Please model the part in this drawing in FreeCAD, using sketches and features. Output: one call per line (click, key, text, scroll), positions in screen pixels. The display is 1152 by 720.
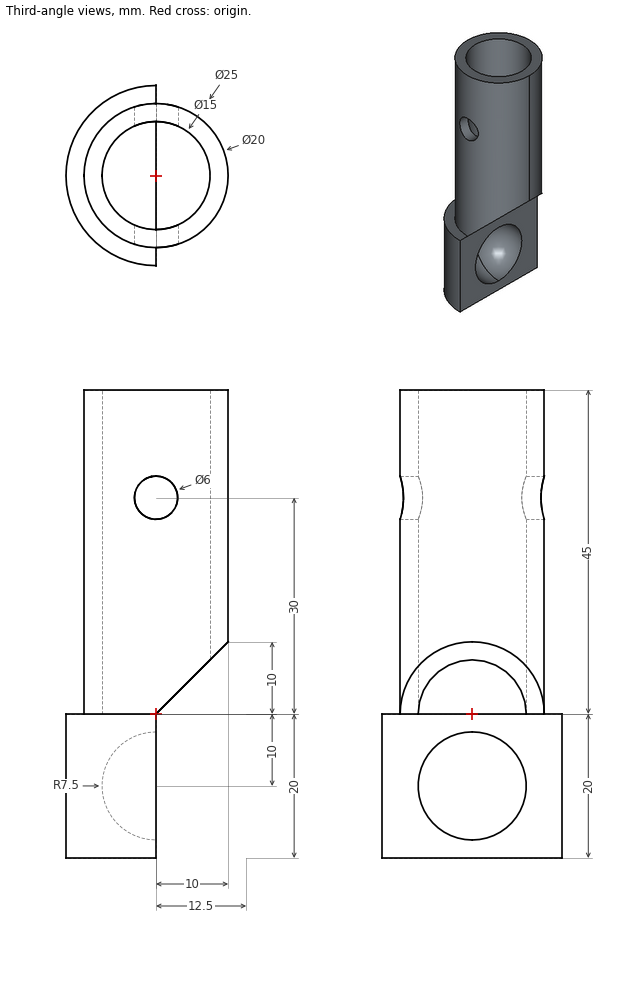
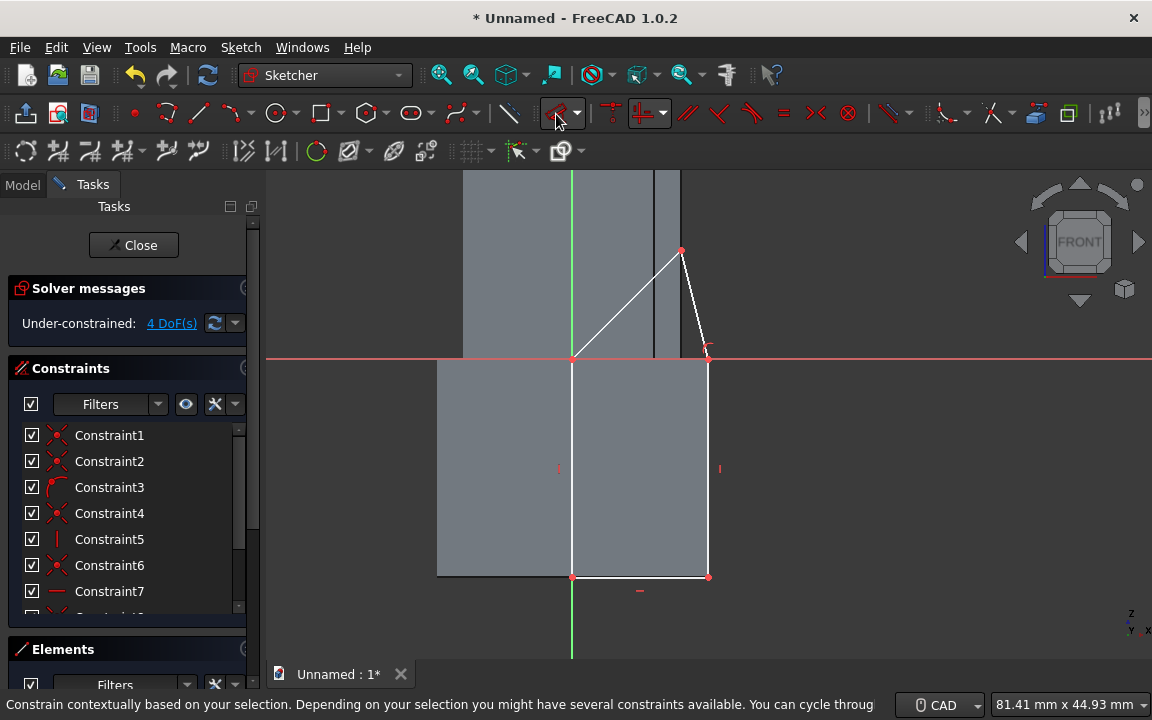
click(708, 425)
click(742, 469)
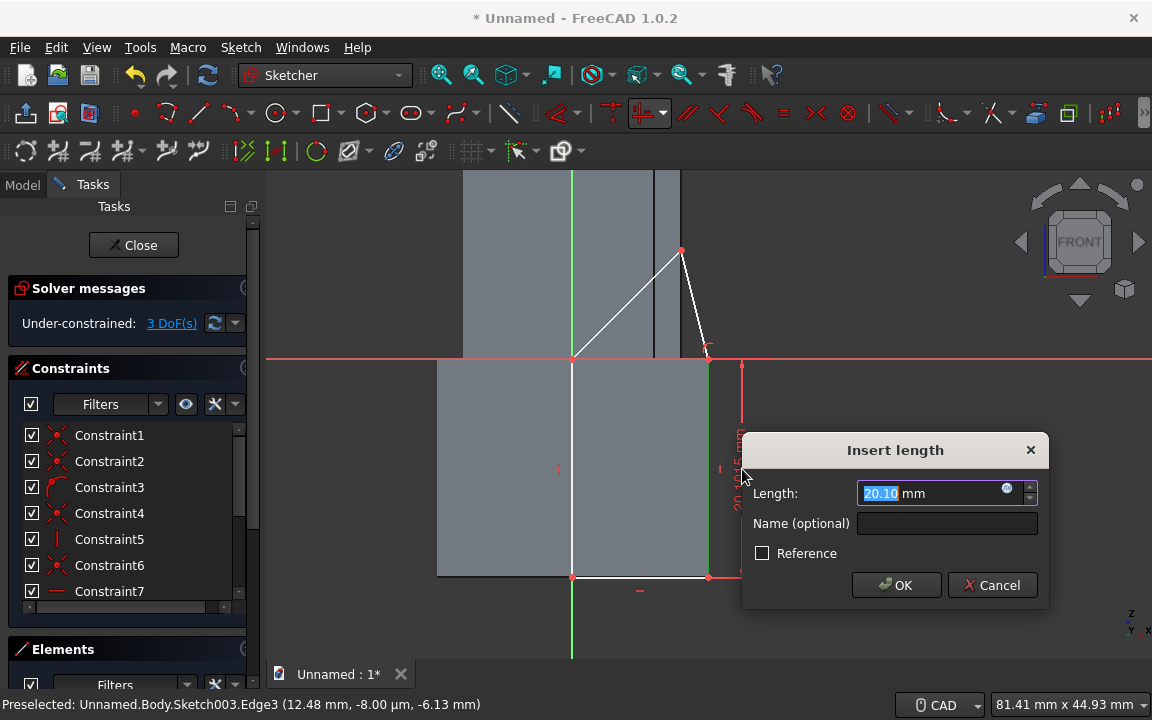
text(20)
key(Return)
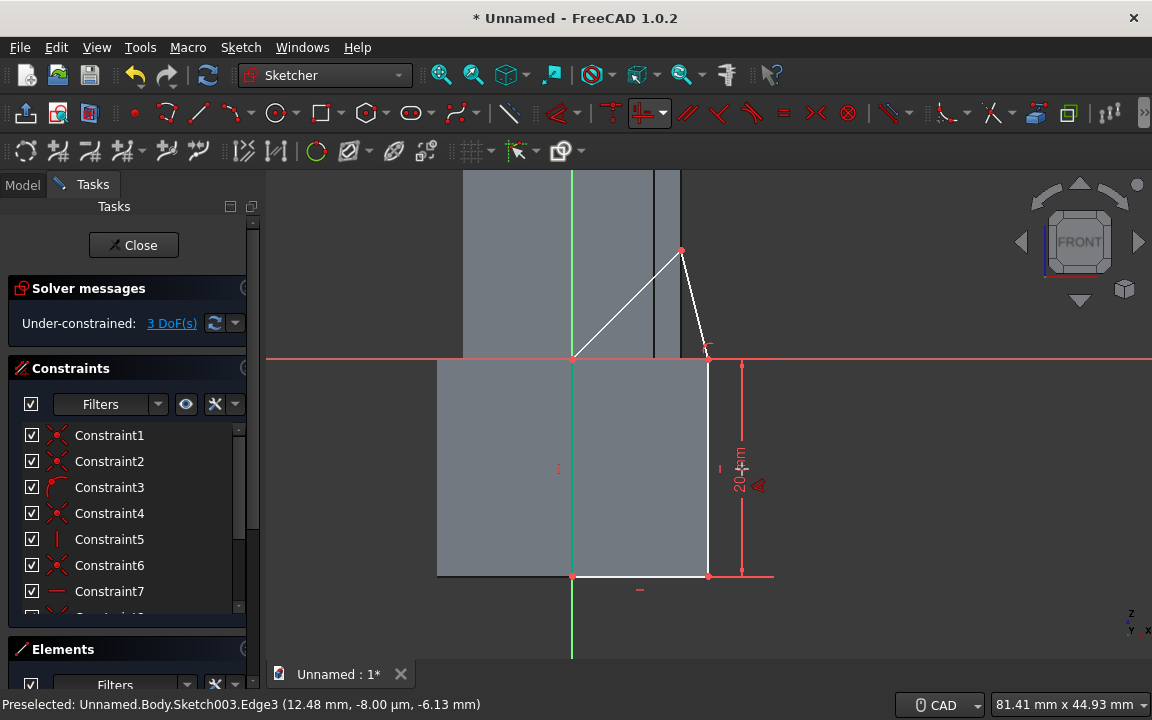
click(681, 251)
click(627, 217)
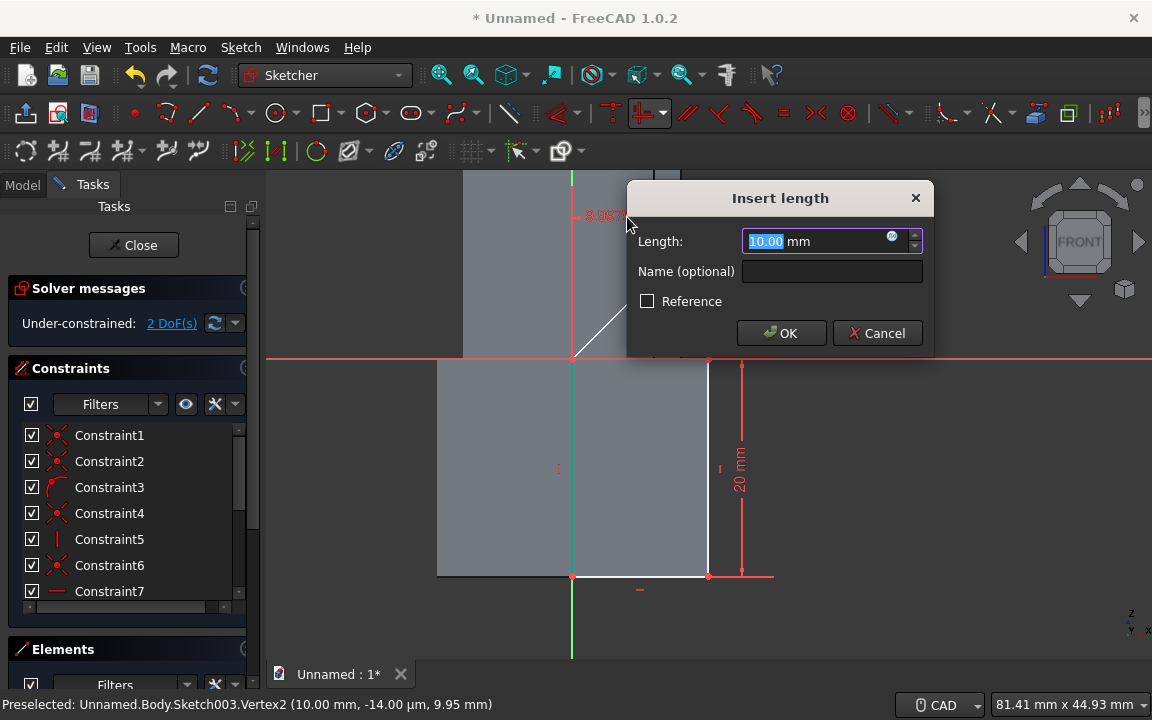
text(10)
key(Return)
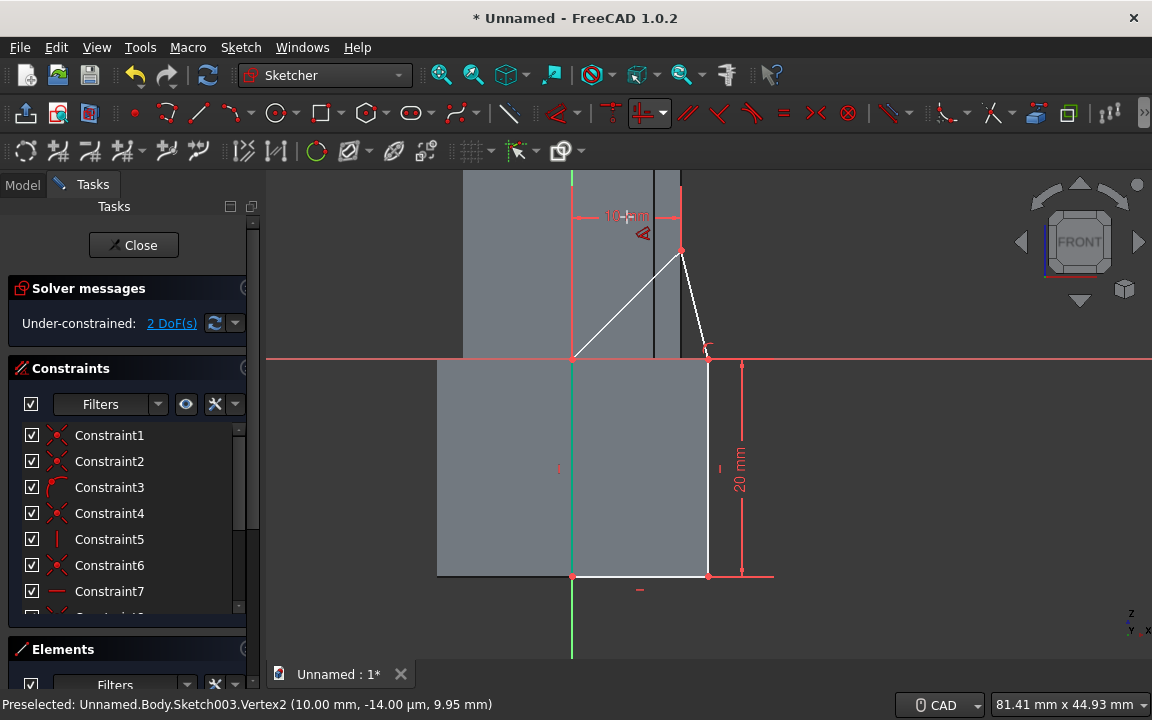
click(681, 251)
click(538, 305)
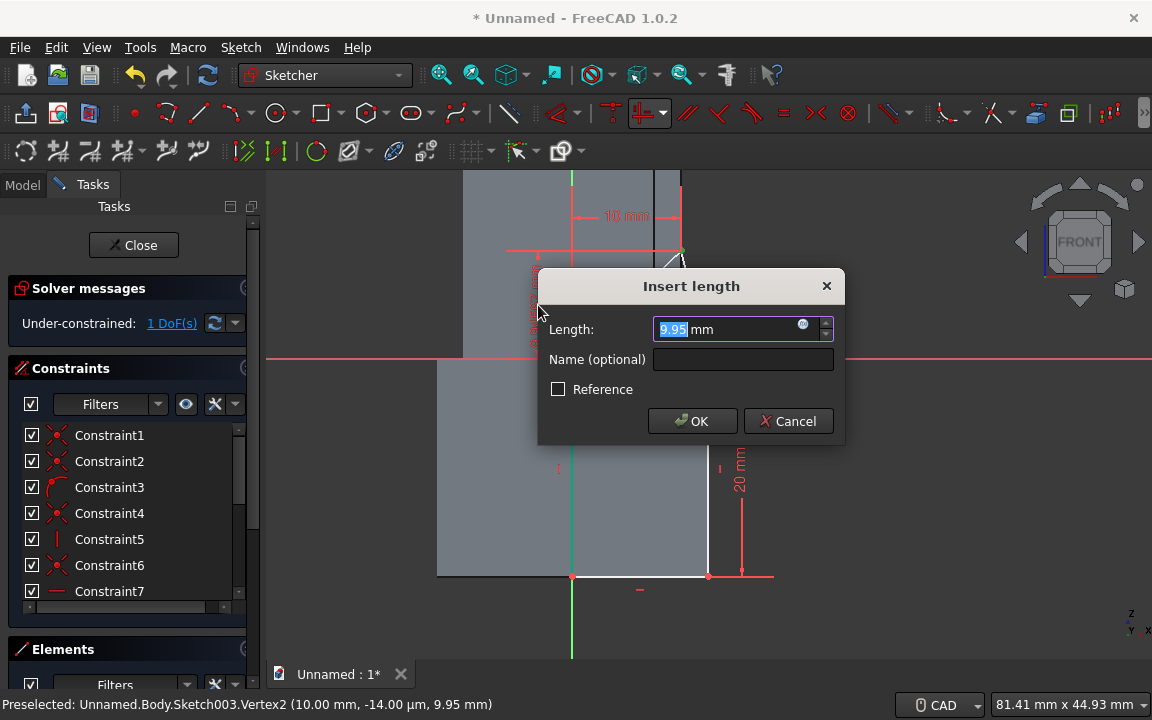
text(10)
key(Return)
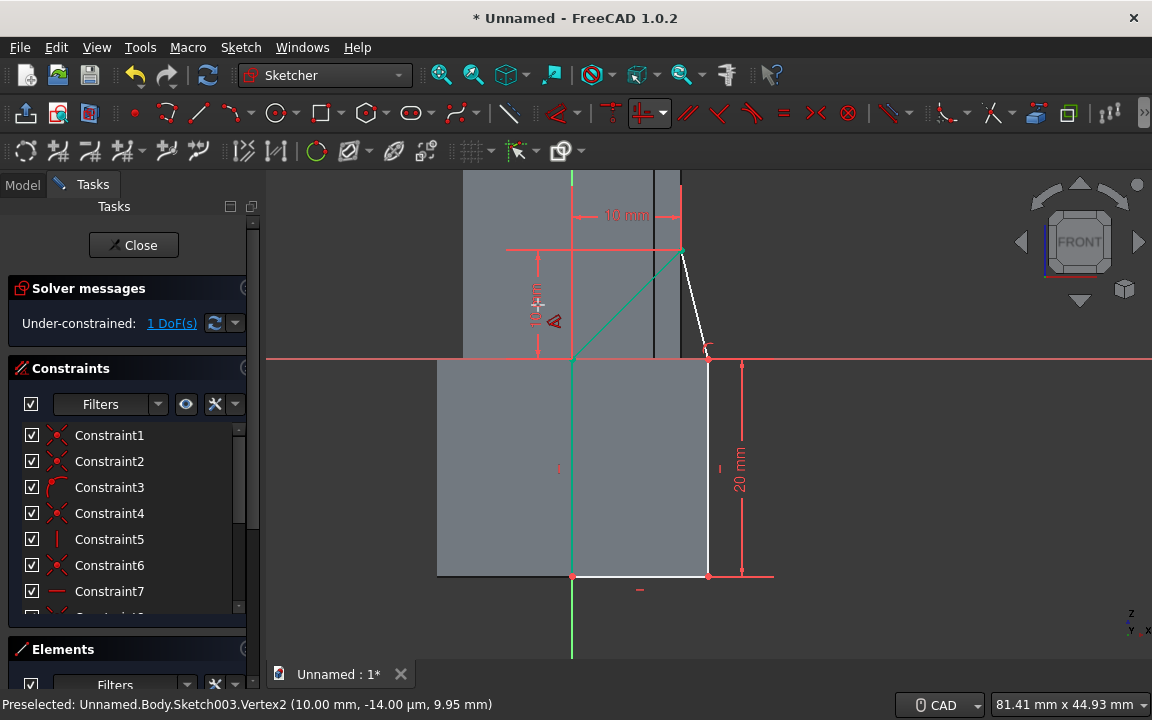
click(667, 577)
click(640, 611)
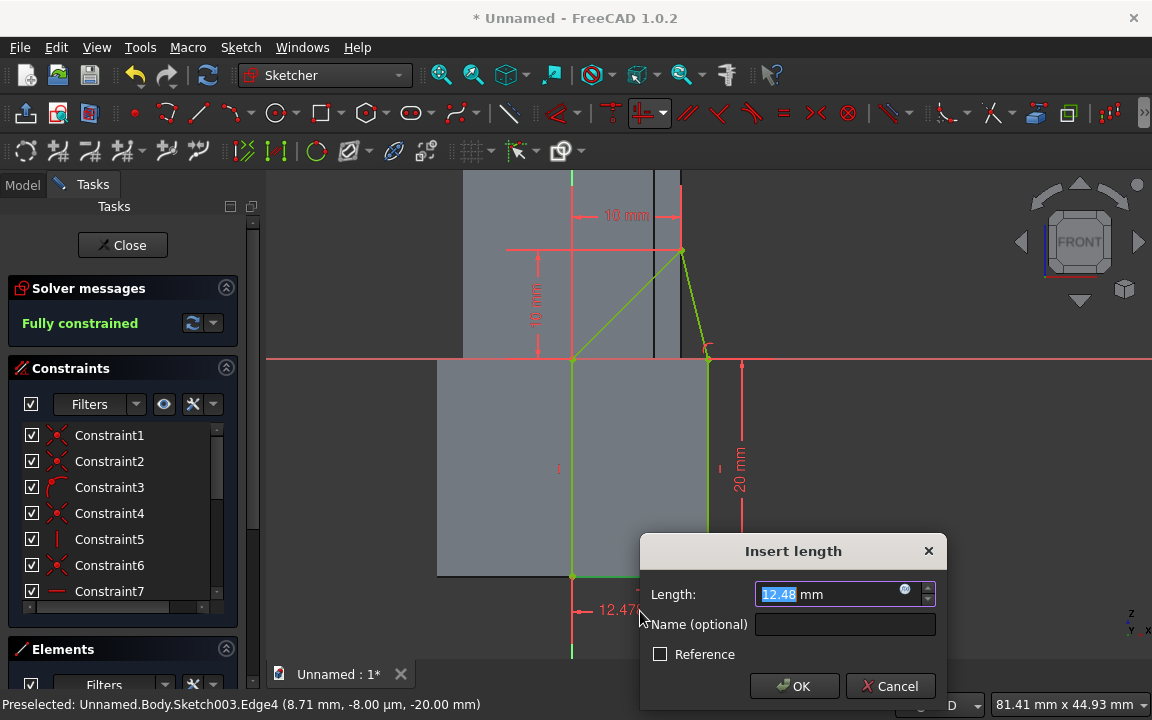
text(12.5)
key(Return)
key(Escape)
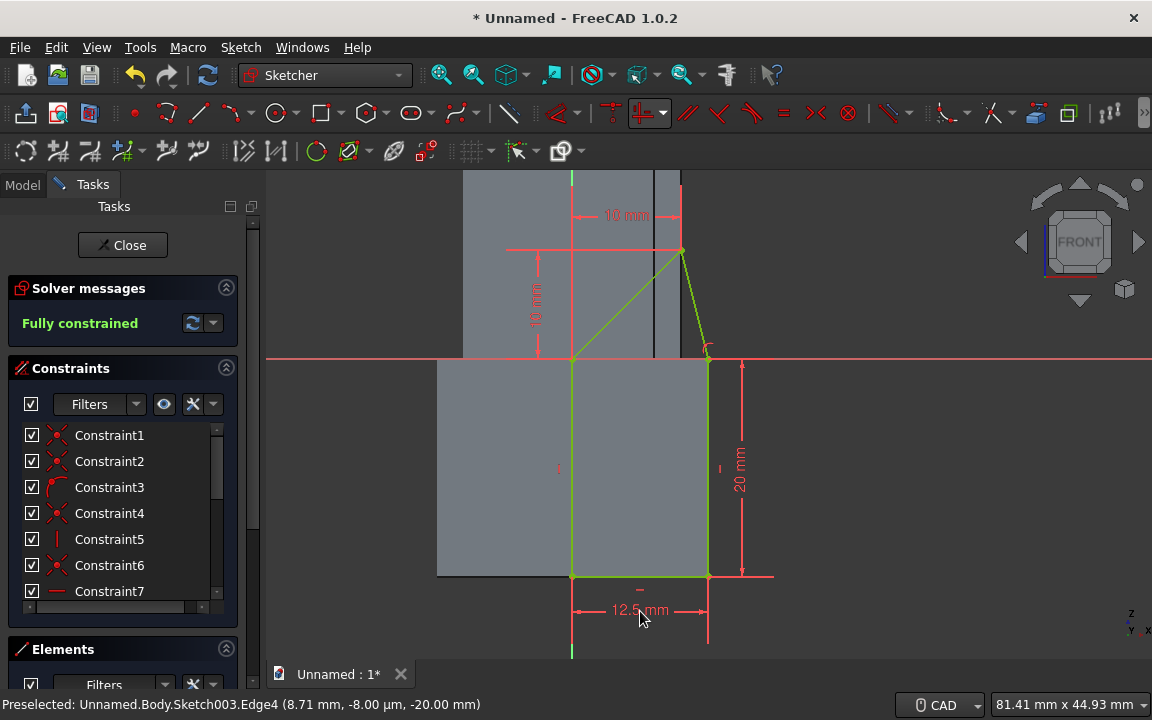
click(123, 245)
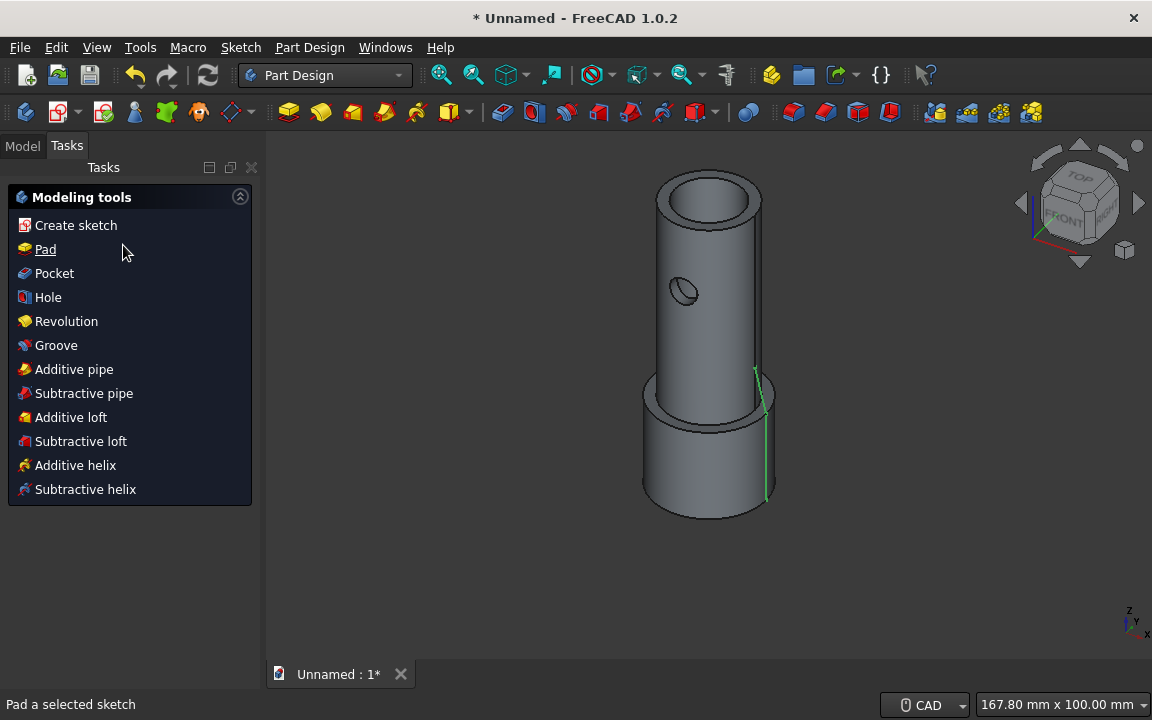
click(504, 112)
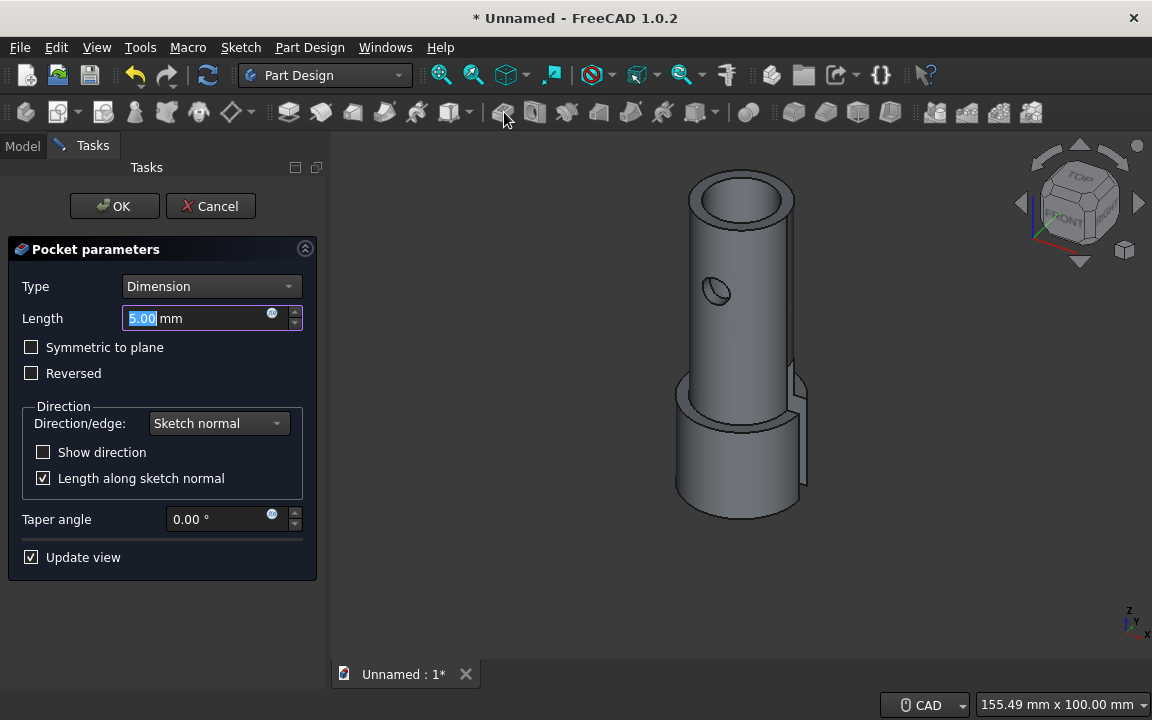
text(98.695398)
key(Tab)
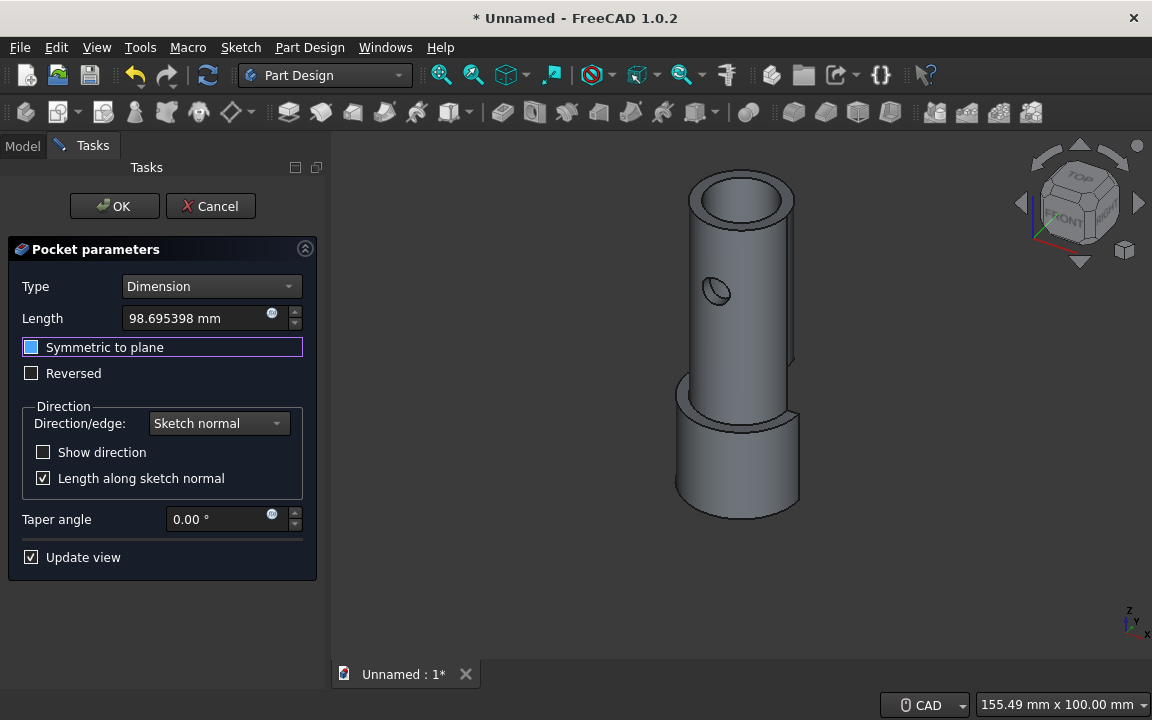
click(30, 347)